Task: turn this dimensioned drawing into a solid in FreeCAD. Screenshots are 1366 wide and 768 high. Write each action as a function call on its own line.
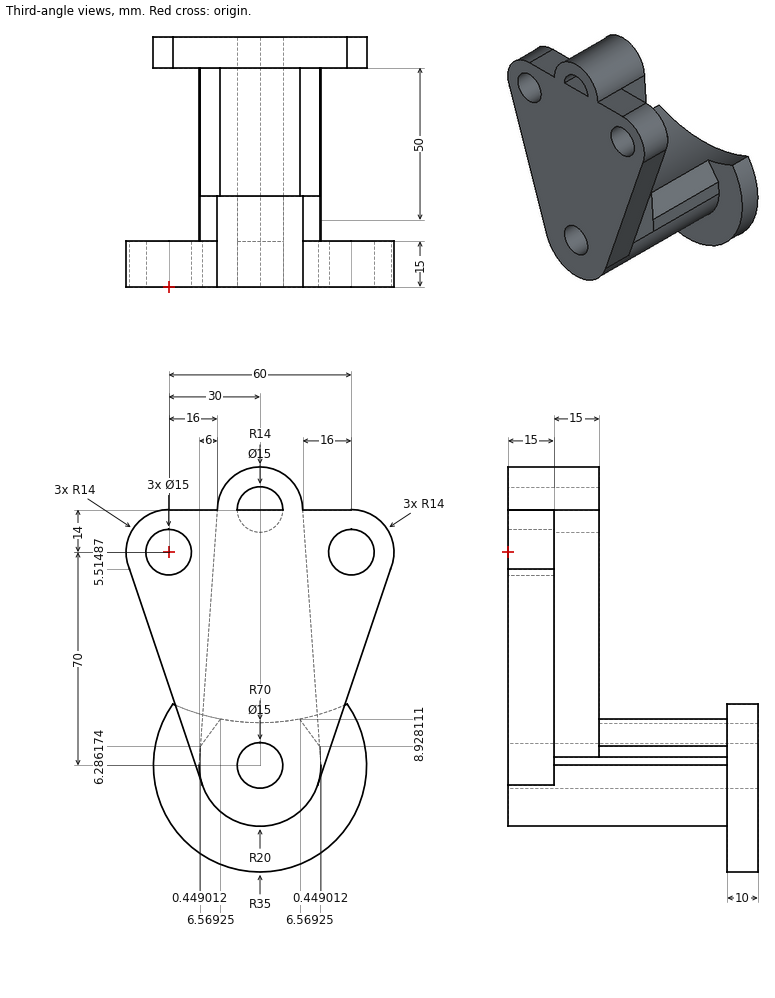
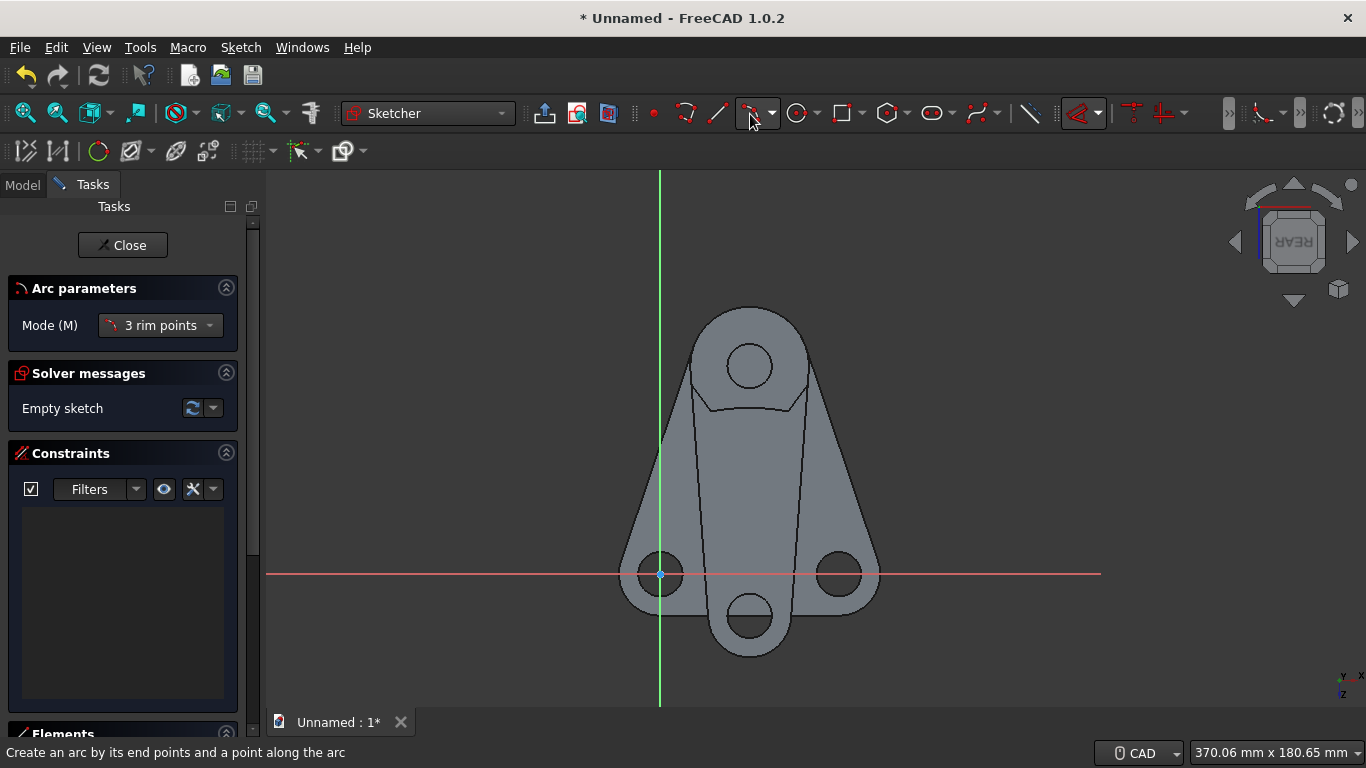
scroll(665, 426, up, 7)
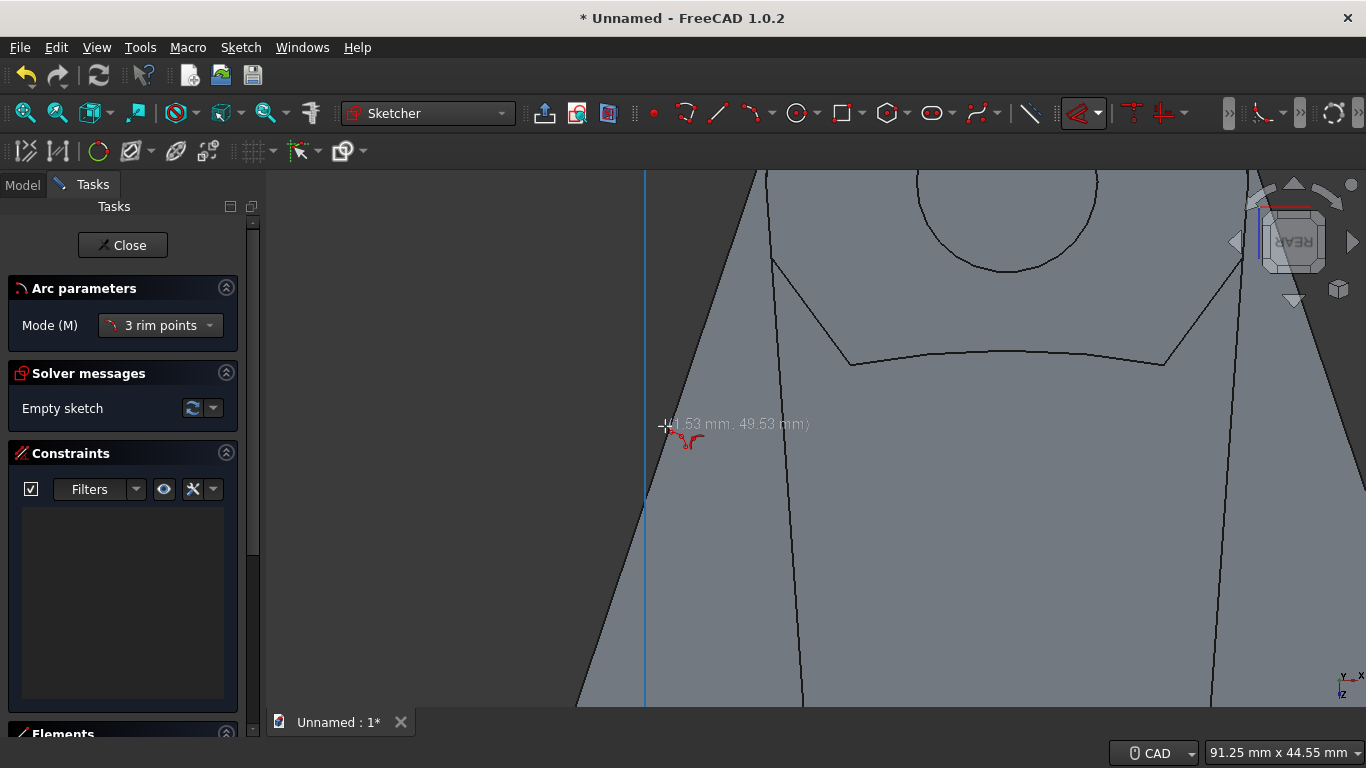
click(662, 424)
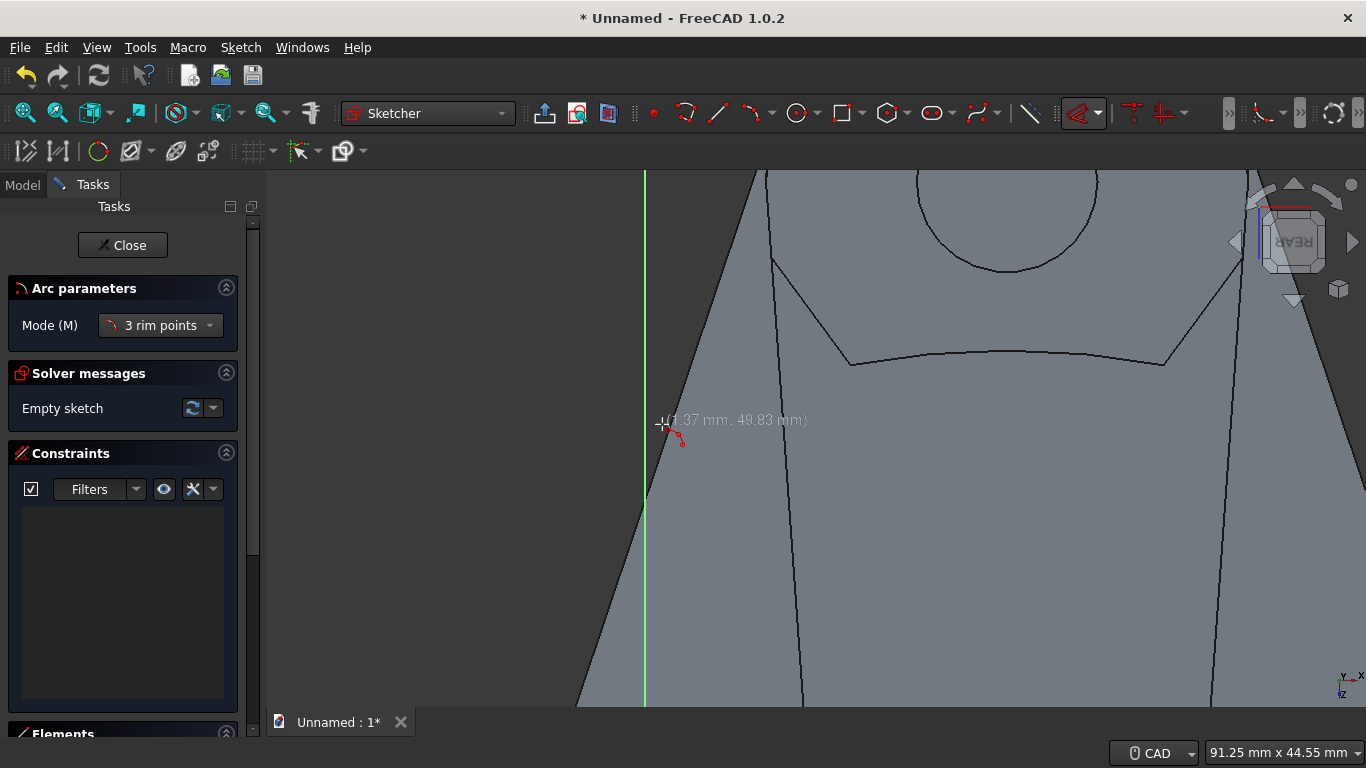
scroll(665, 453, down, 7)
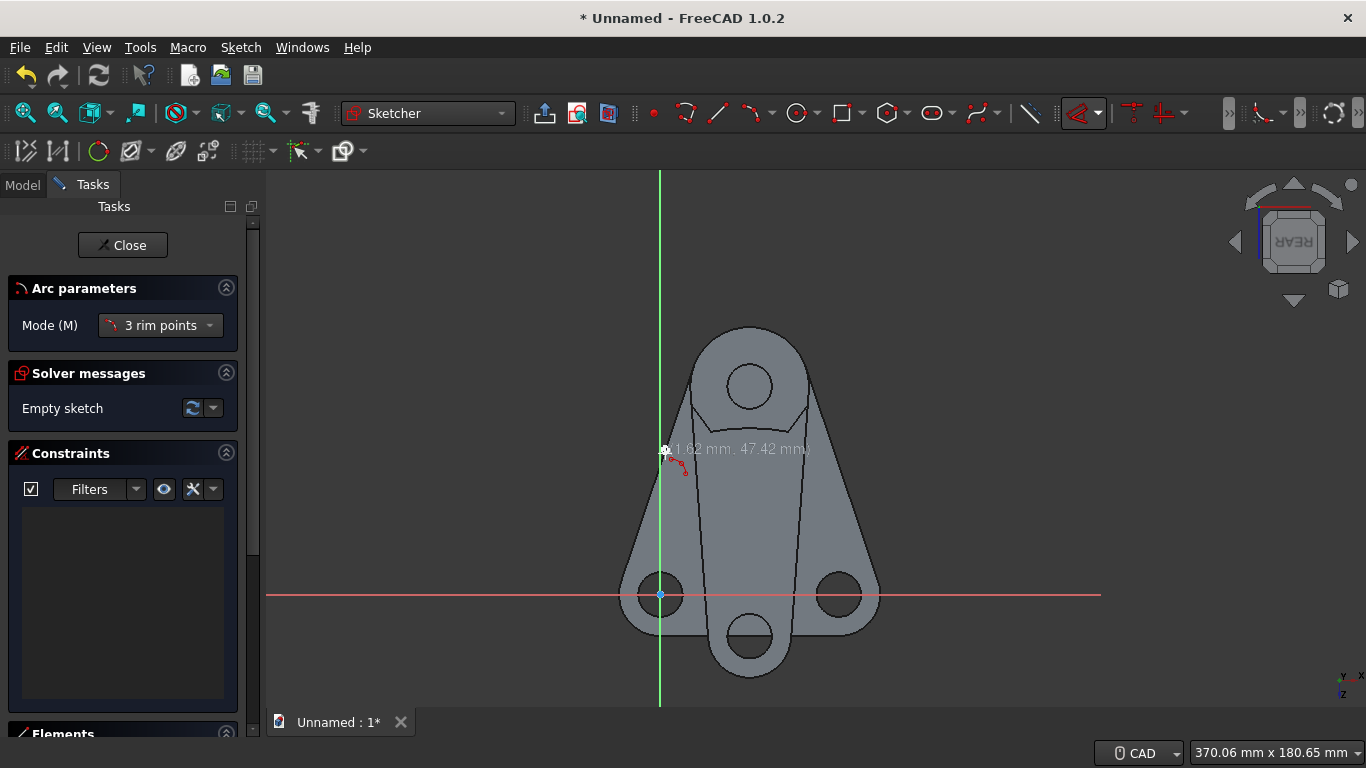
click(835, 446)
click(750, 428)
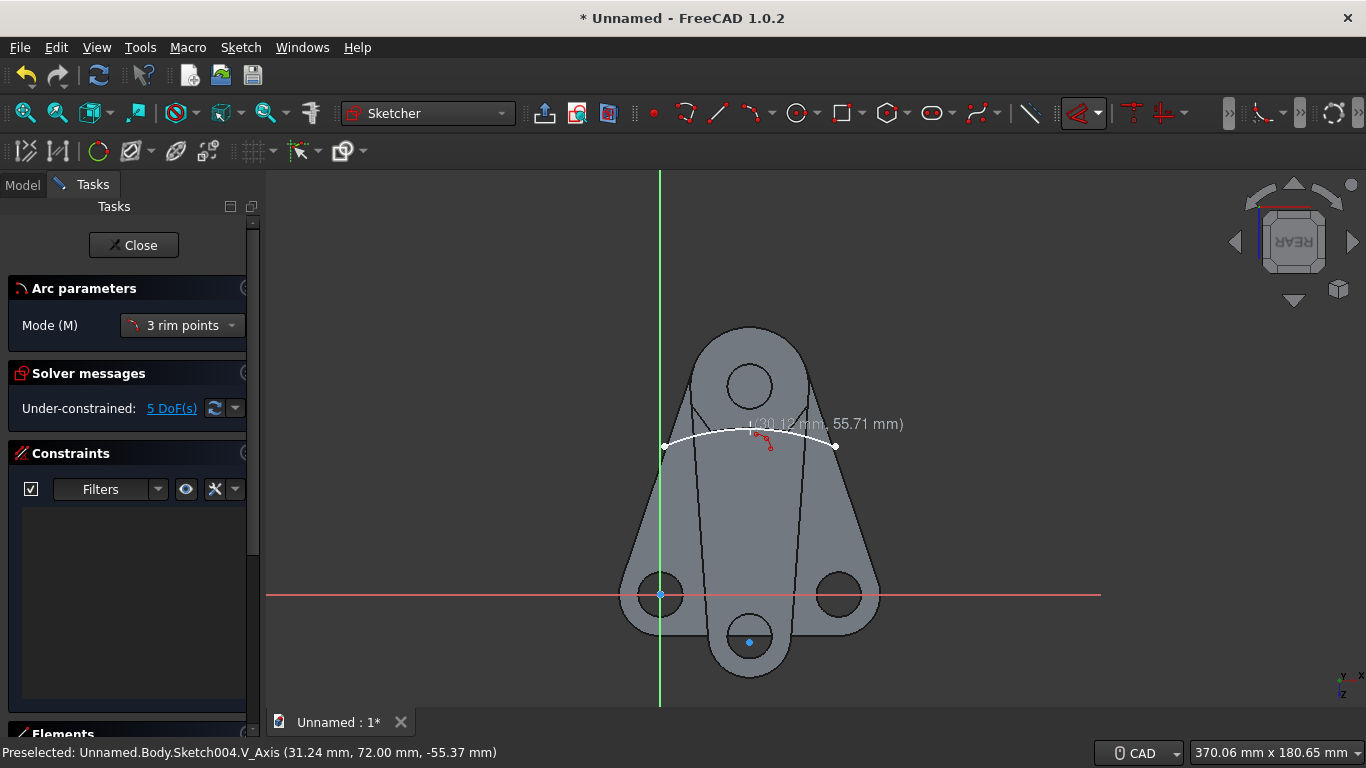
click(835, 447)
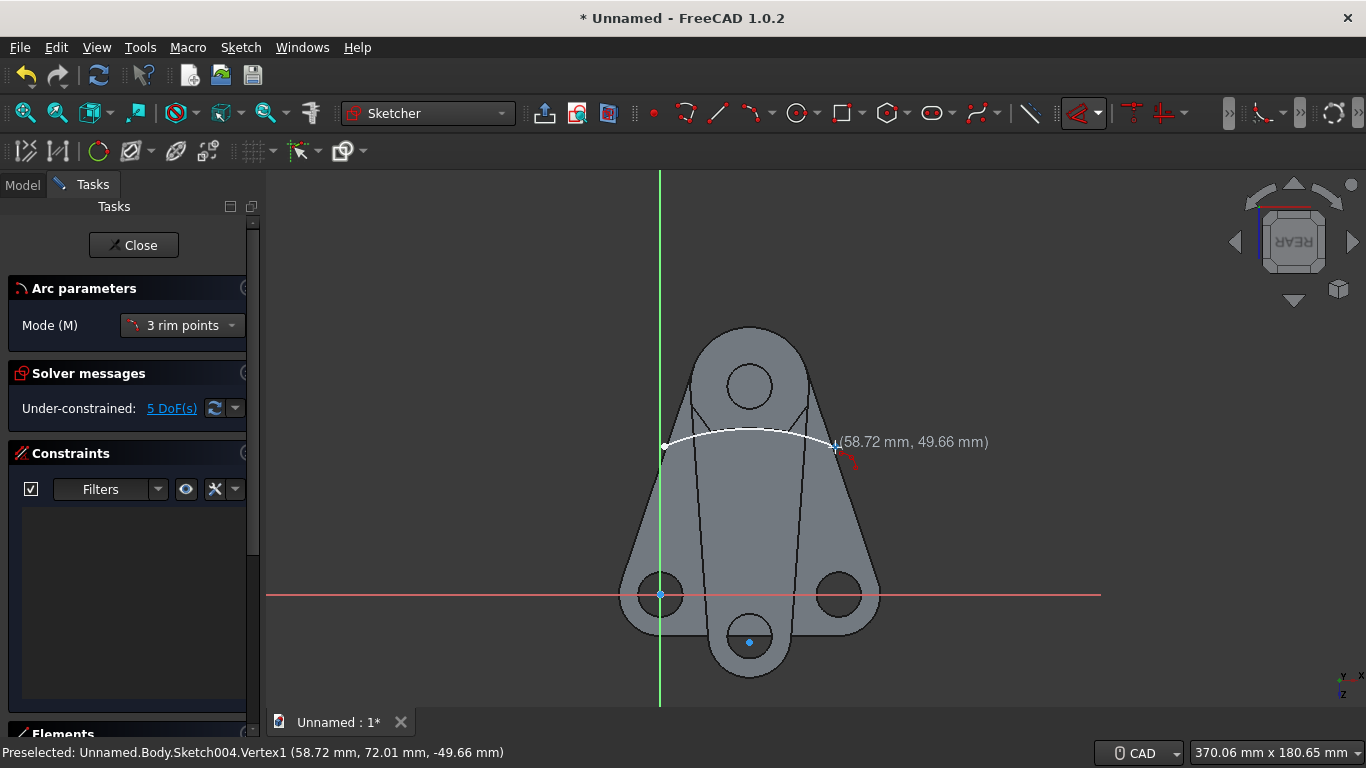
scroll(665, 446, up, 7)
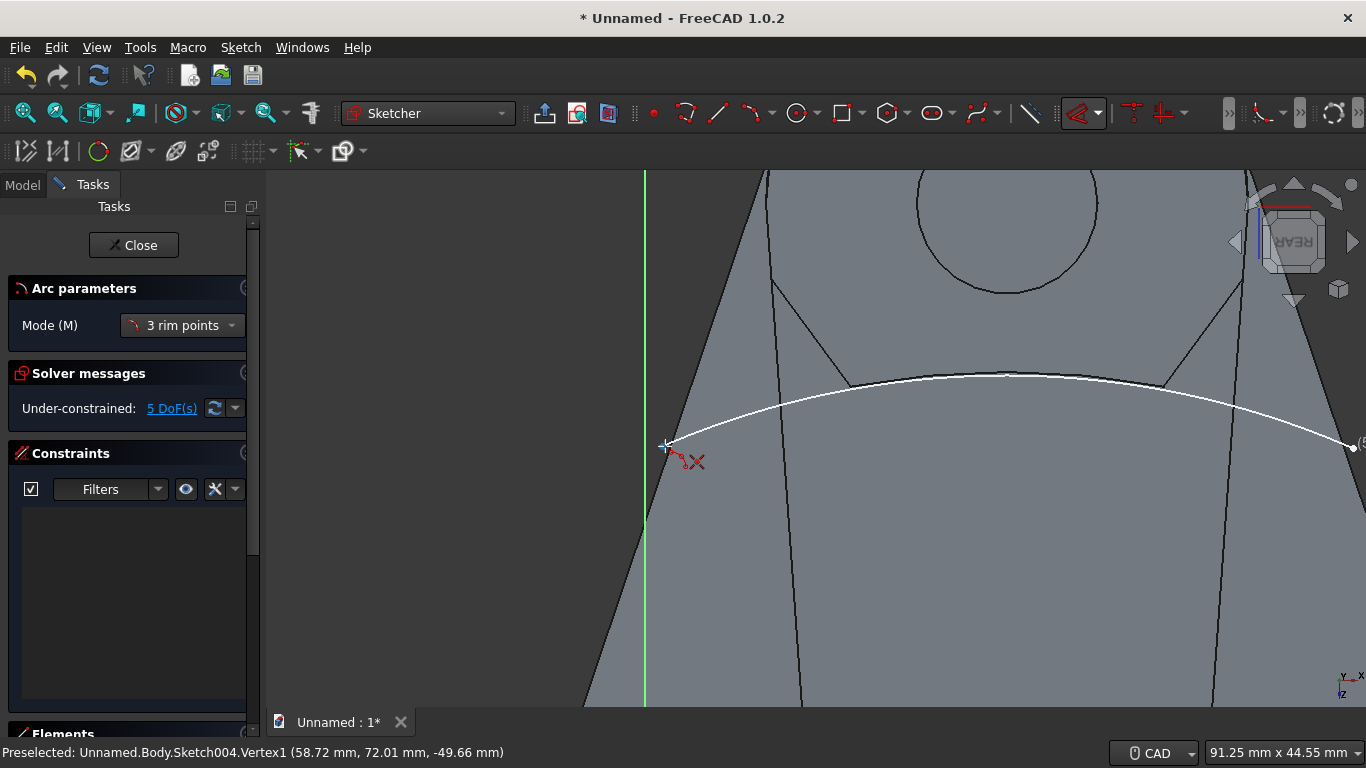
click(662, 446)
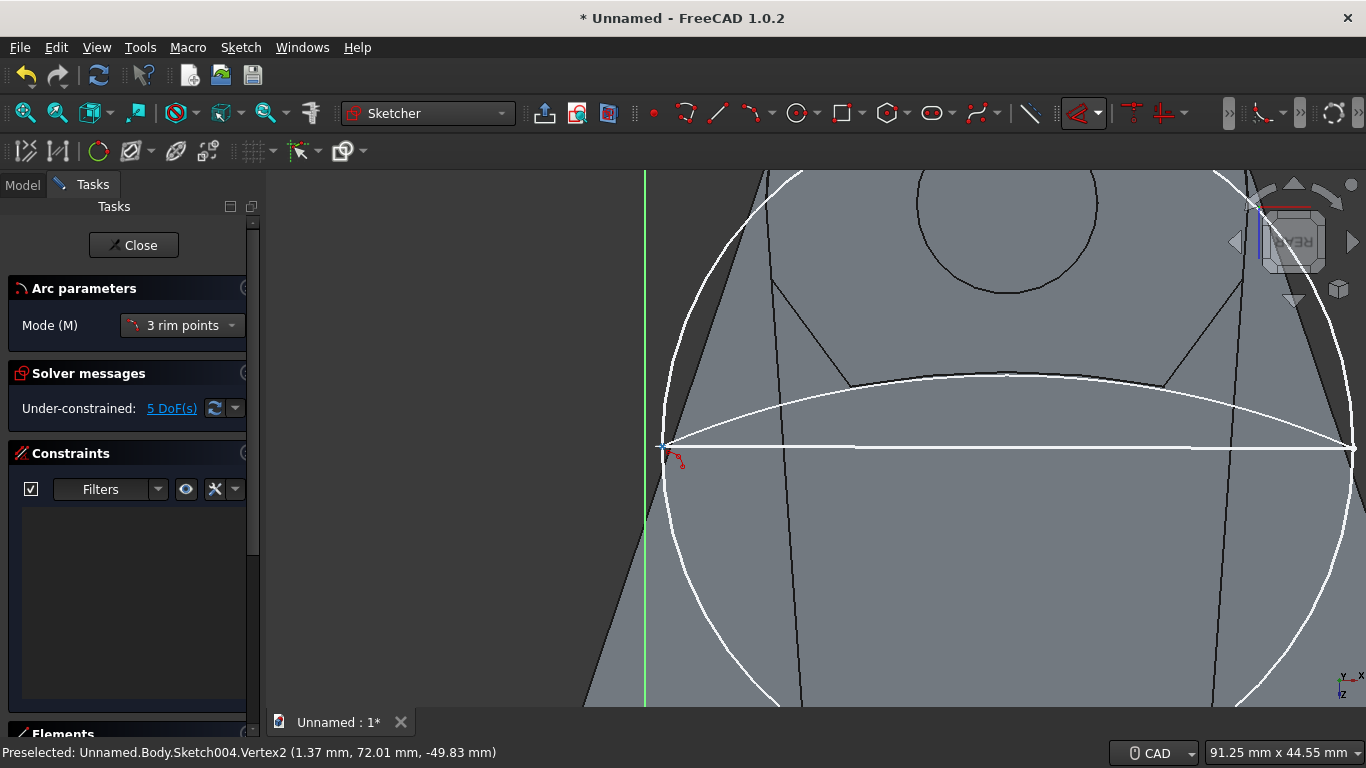
scroll(665, 446, down, 7)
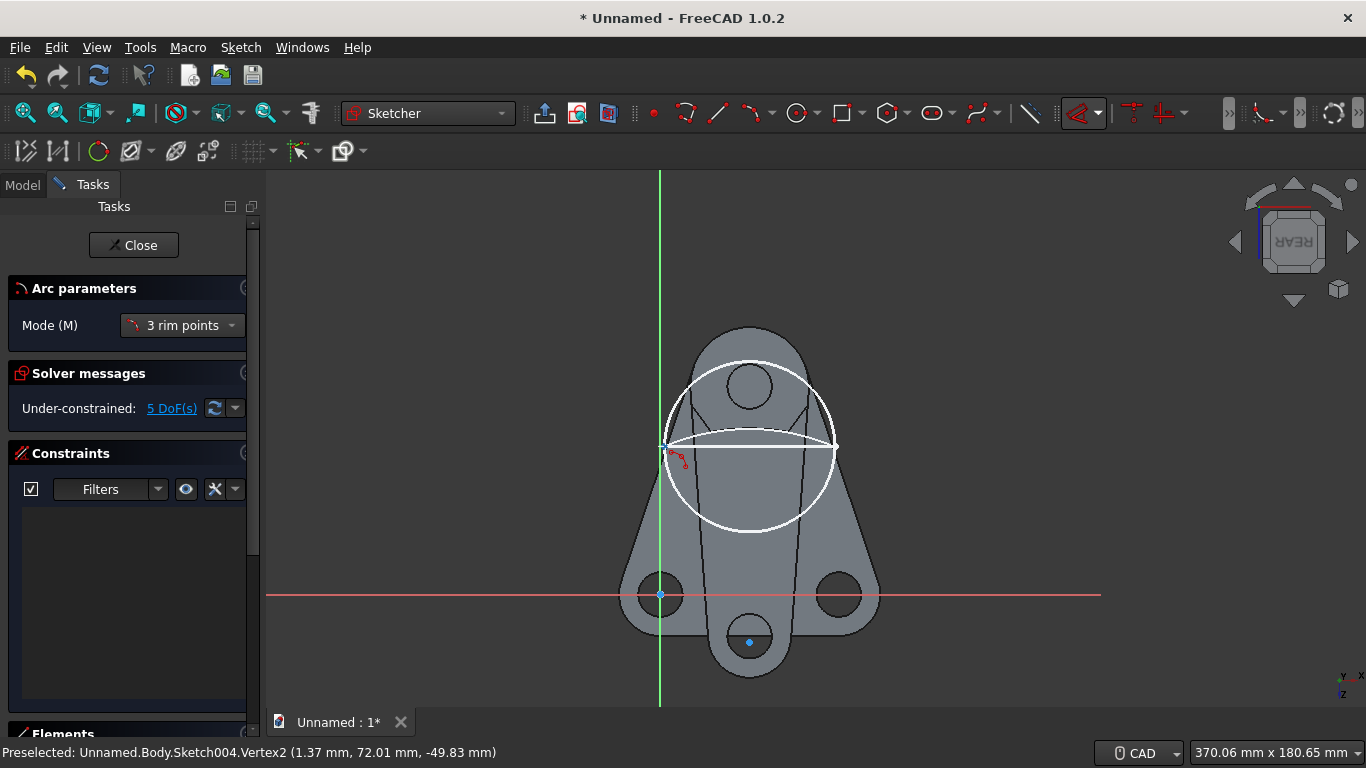
click(750, 282)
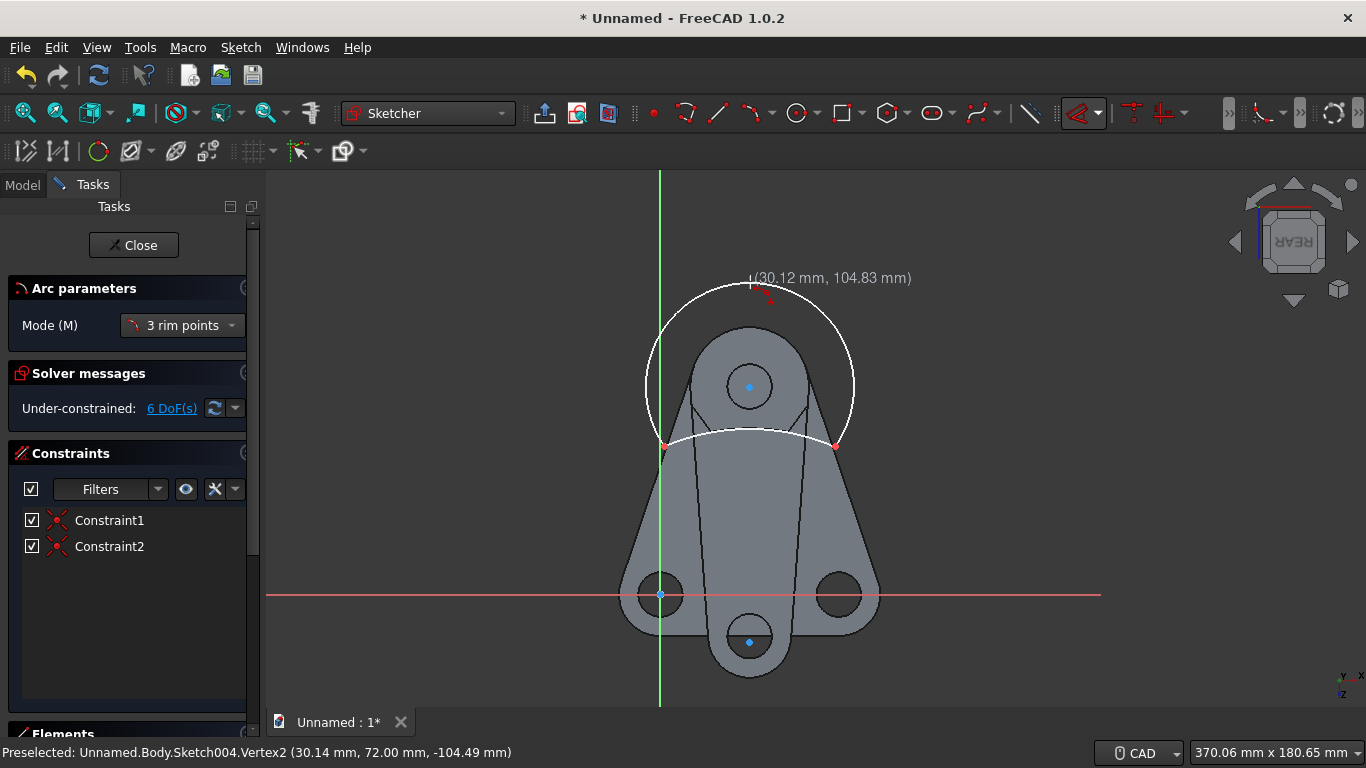
click(798, 114)